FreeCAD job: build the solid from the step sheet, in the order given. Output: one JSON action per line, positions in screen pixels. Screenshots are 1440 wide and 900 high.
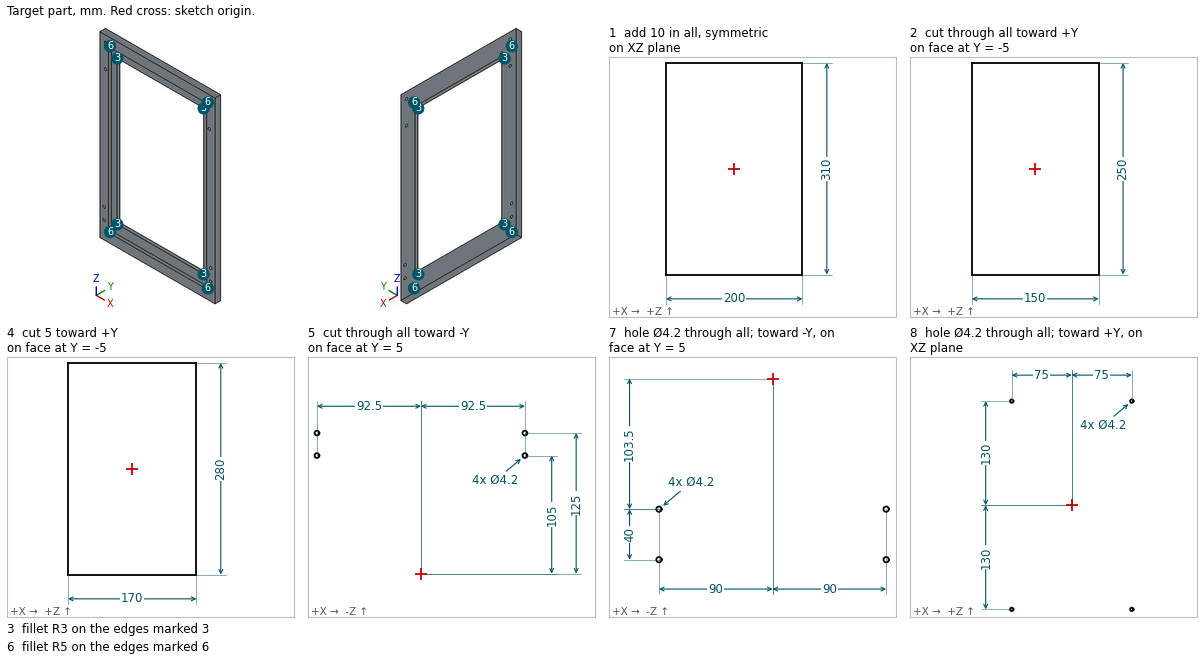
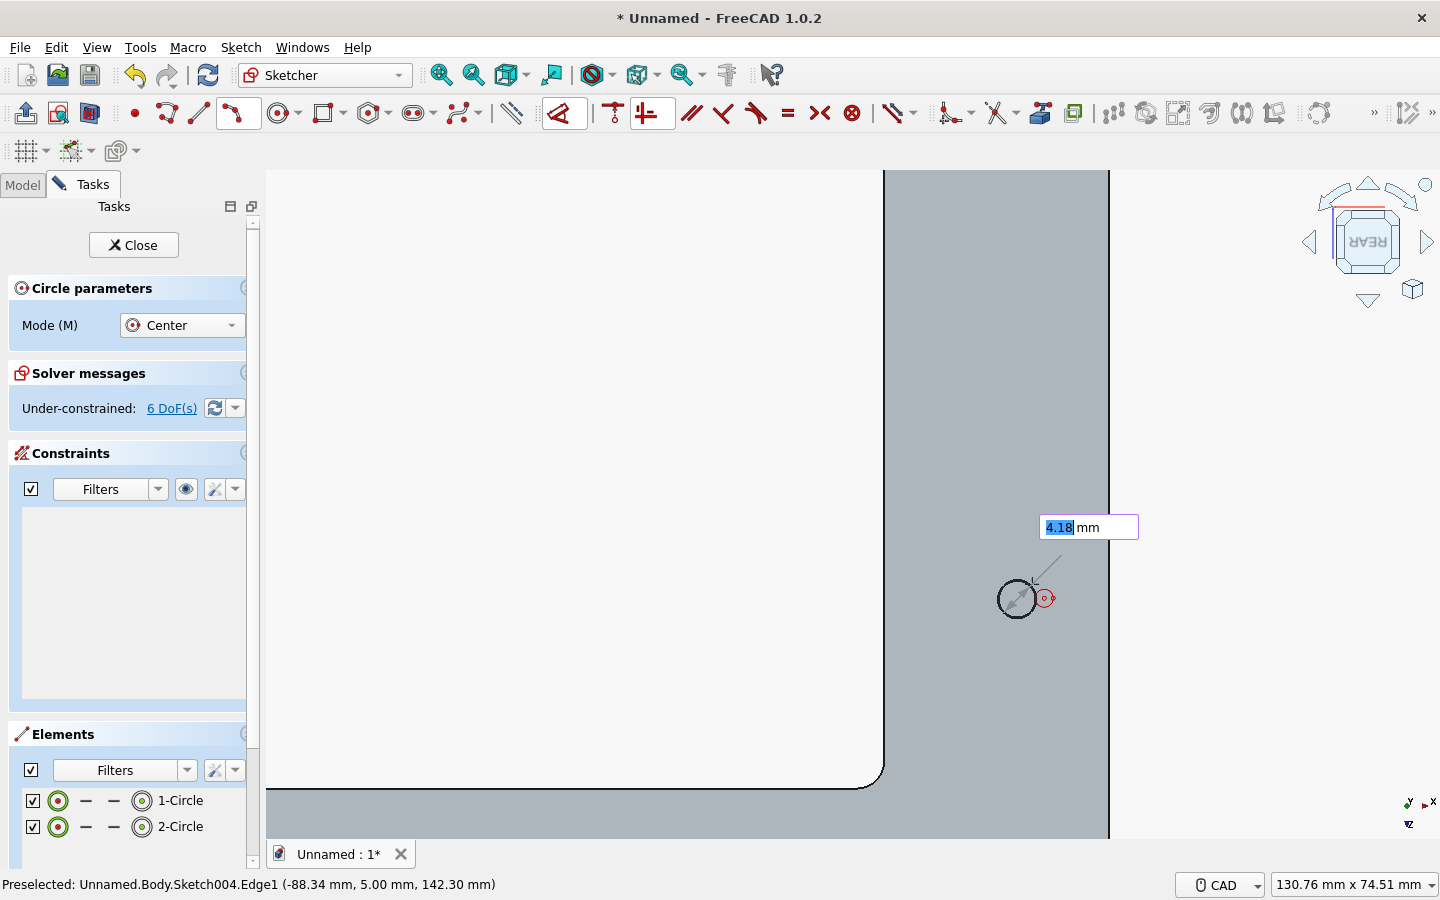
{"action": "left_click", "coordinate": [1032, 582]}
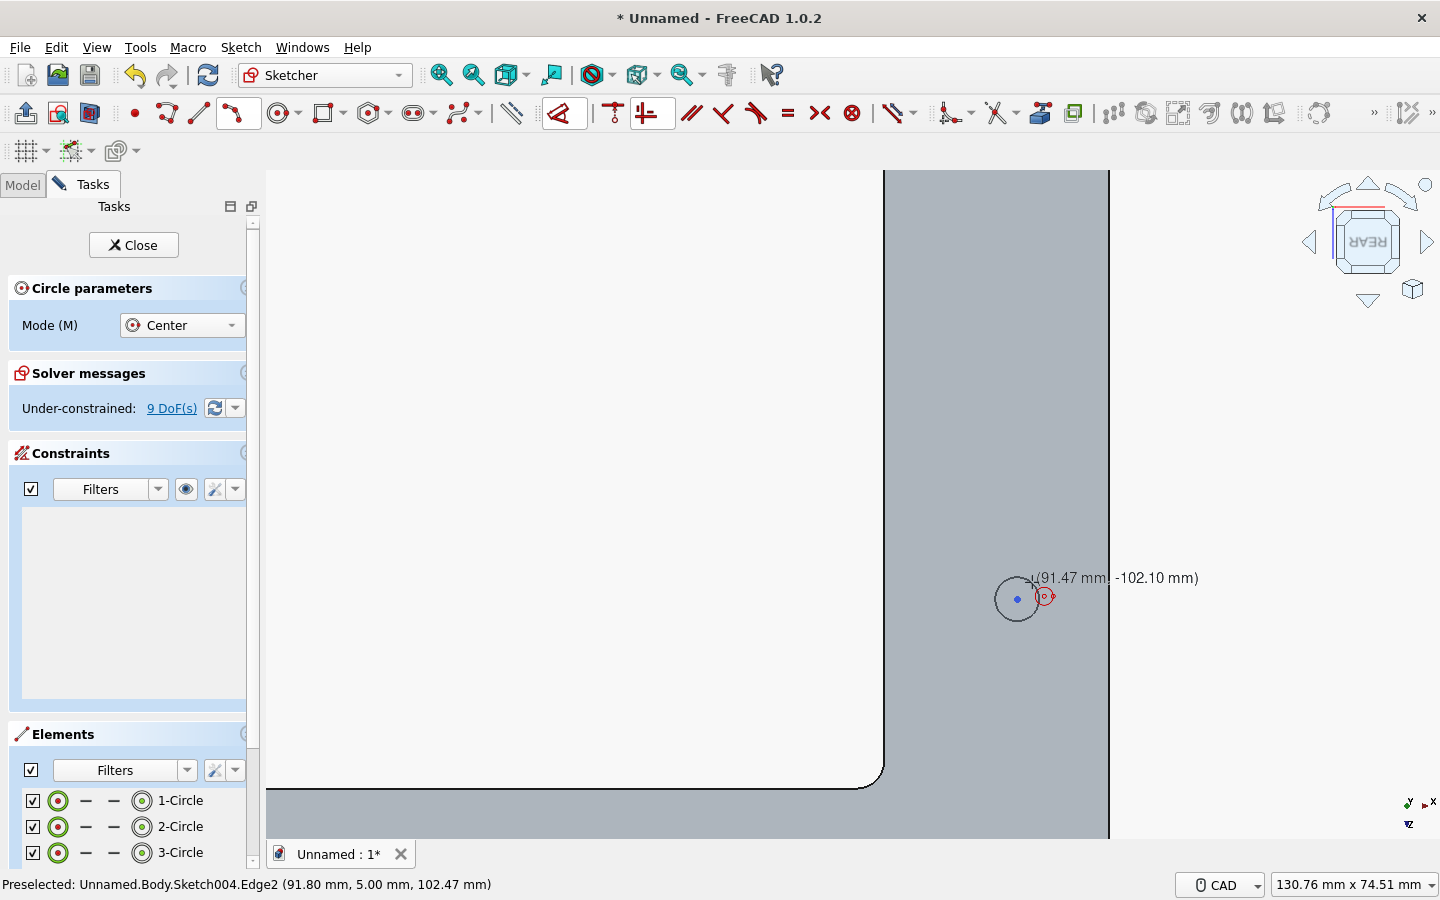
{"action": "scroll", "coordinate": [1032, 584], "scroll_direction": "down", "scroll_amount": 6}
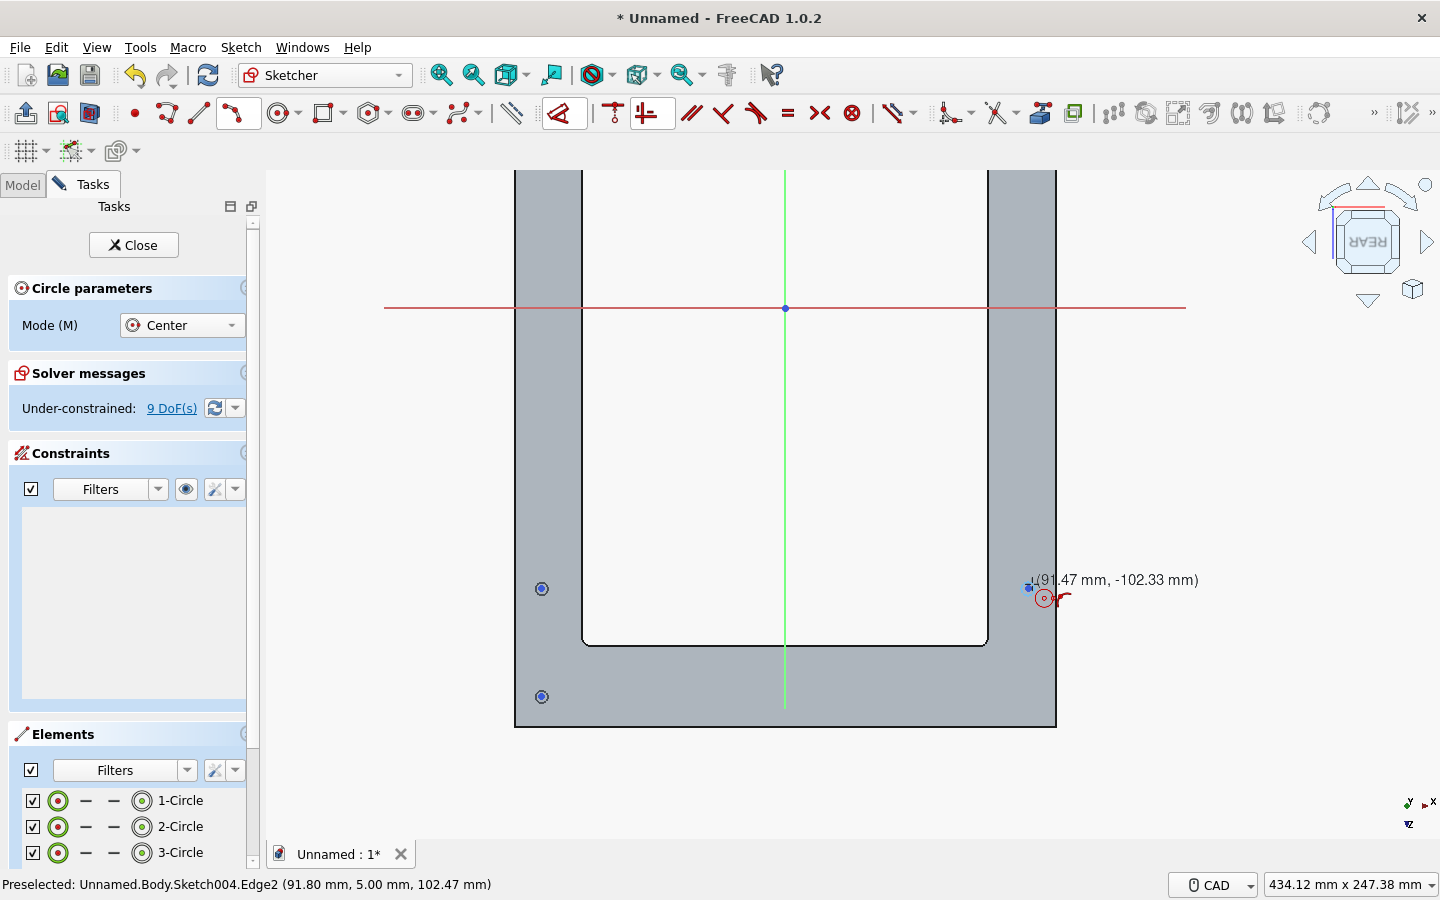
{"action": "scroll", "coordinate": [1028, 696], "scroll_direction": "up", "scroll_amount": 7}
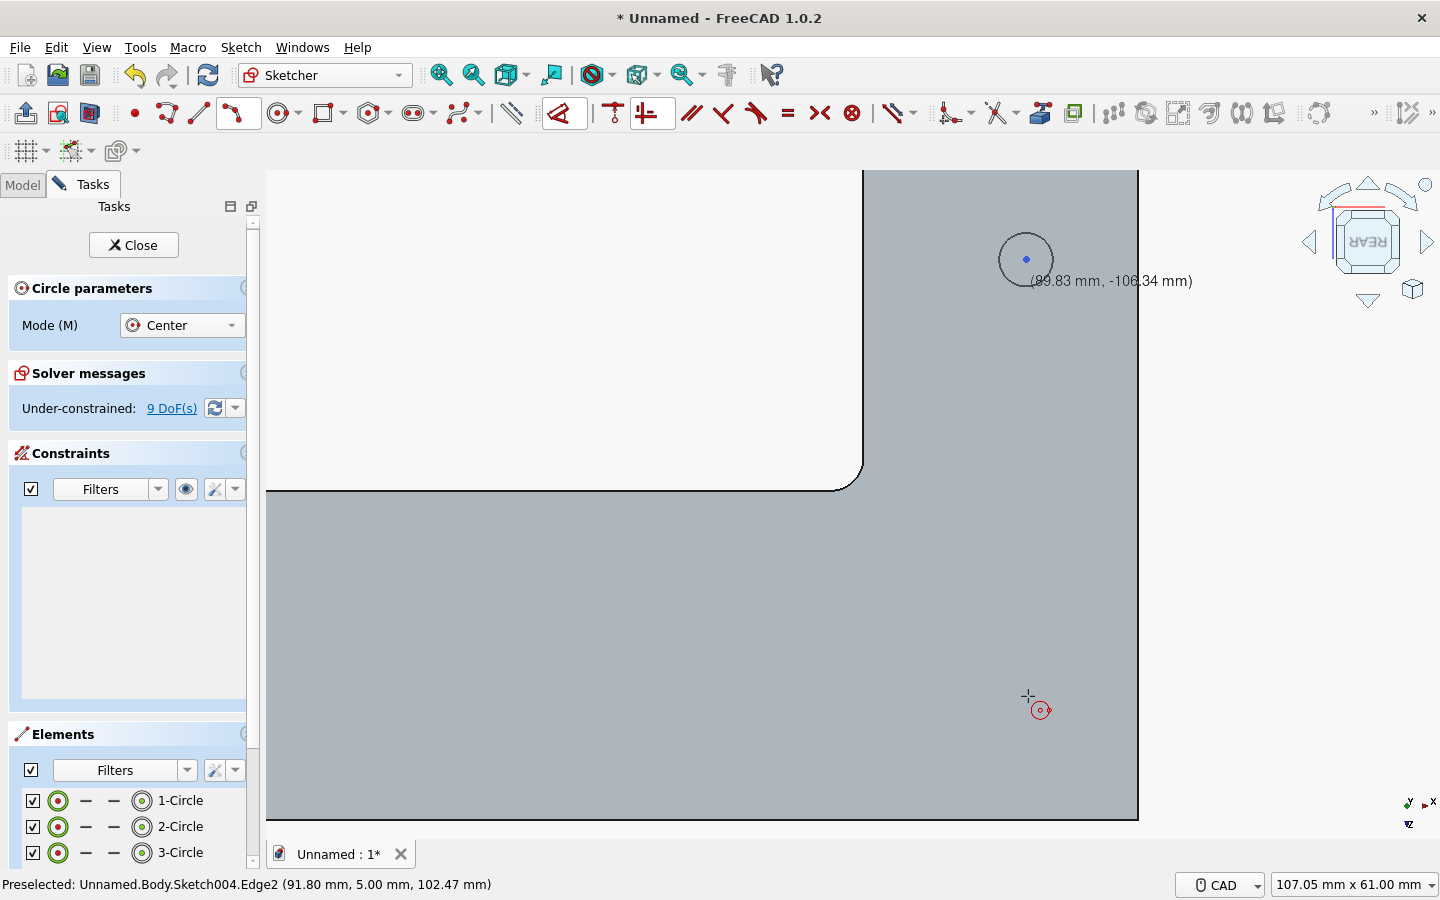
{"action": "scroll", "coordinate": [1028, 696], "scroll_direction": "down", "scroll_amount": 7}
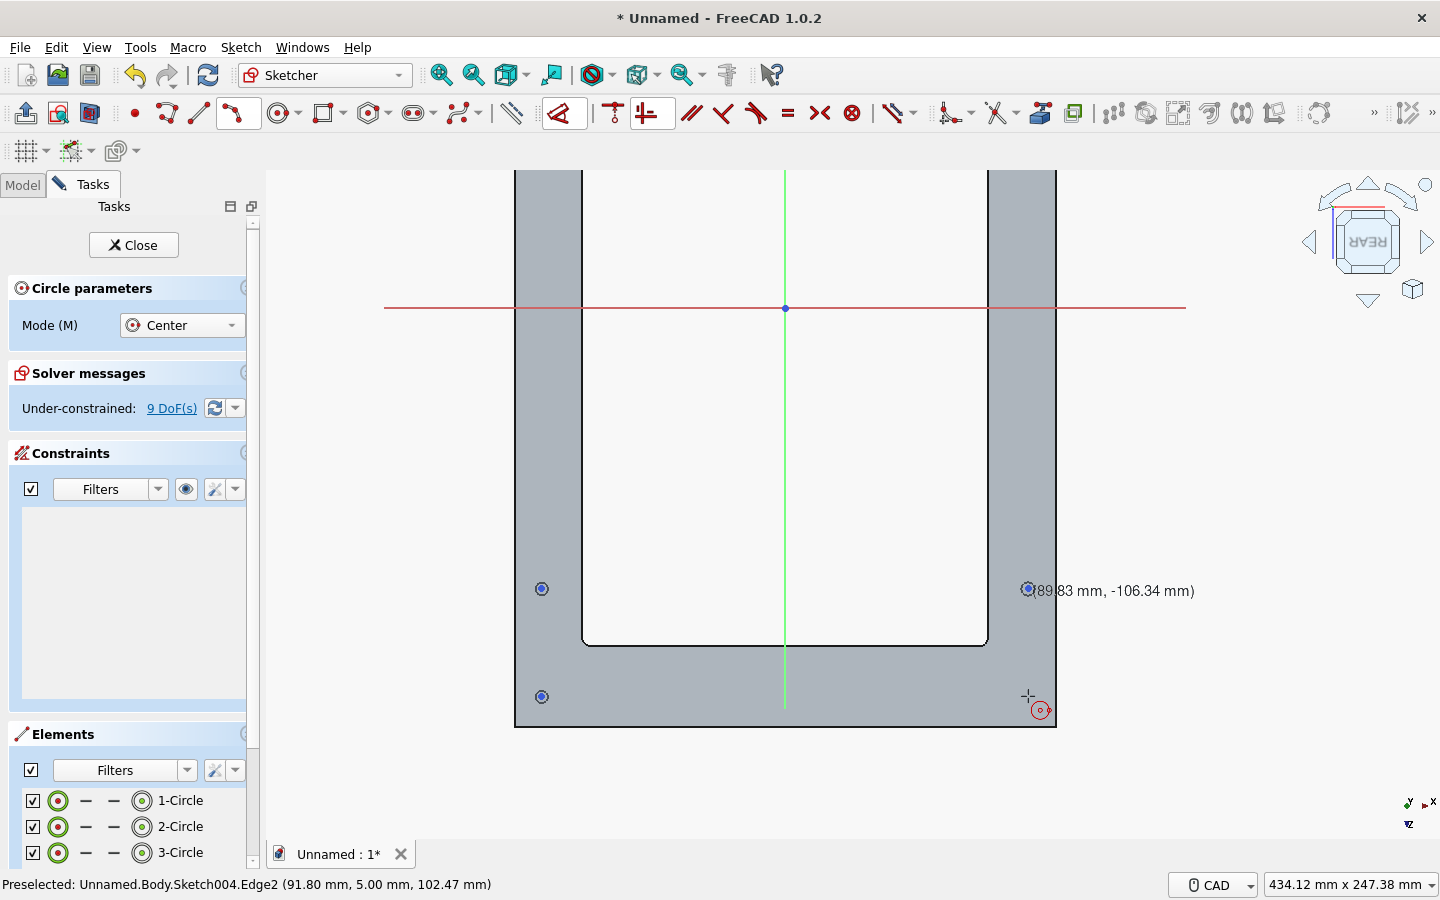
{"action": "left_click", "coordinate": [1028, 696]}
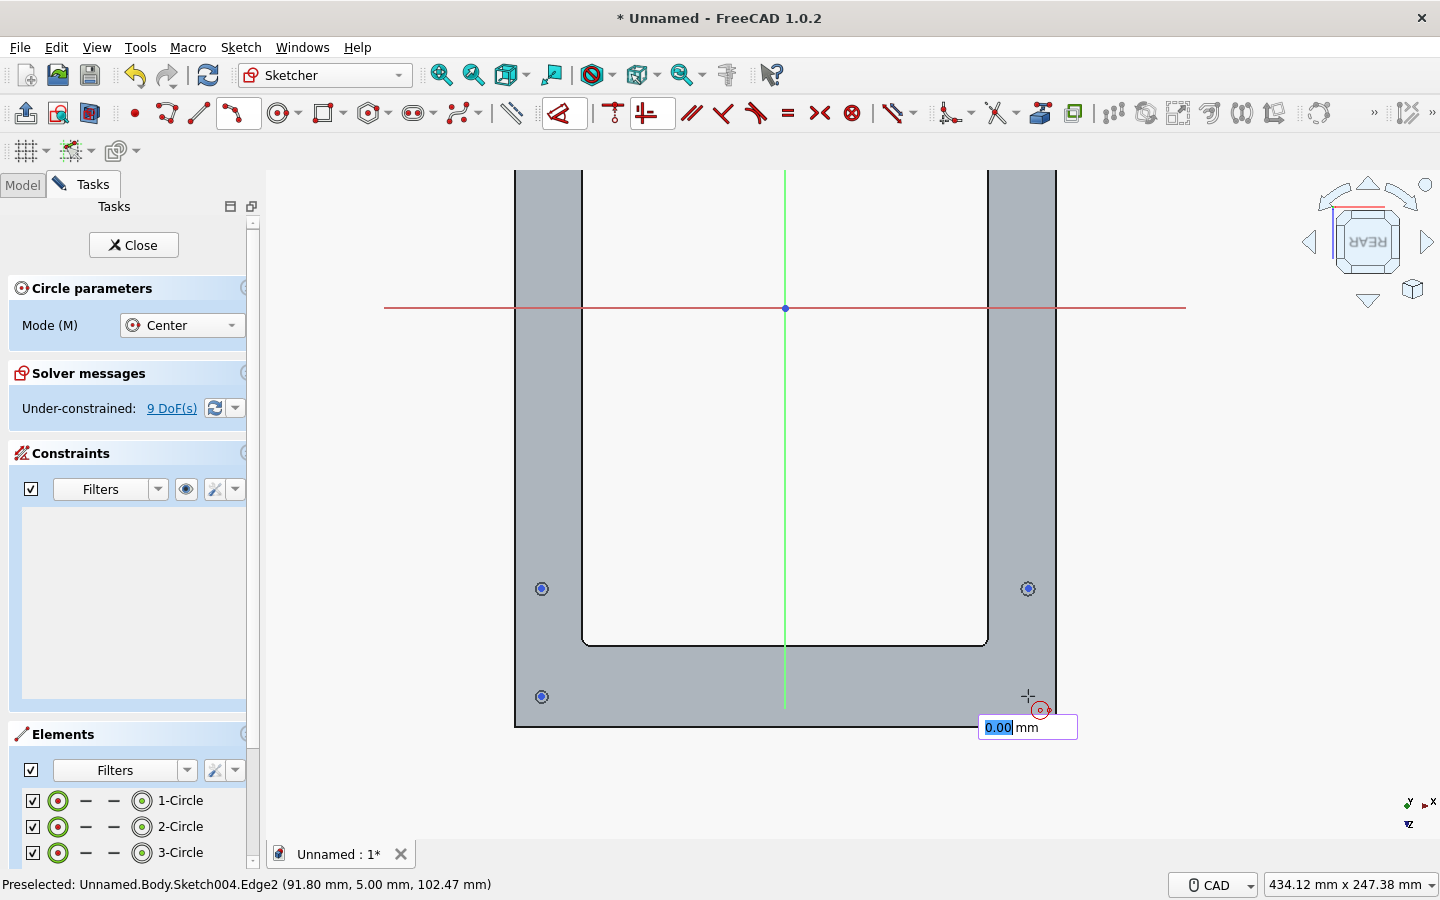
{"action": "scroll", "coordinate": [1032, 692], "scroll_direction": "up", "scroll_amount": 6}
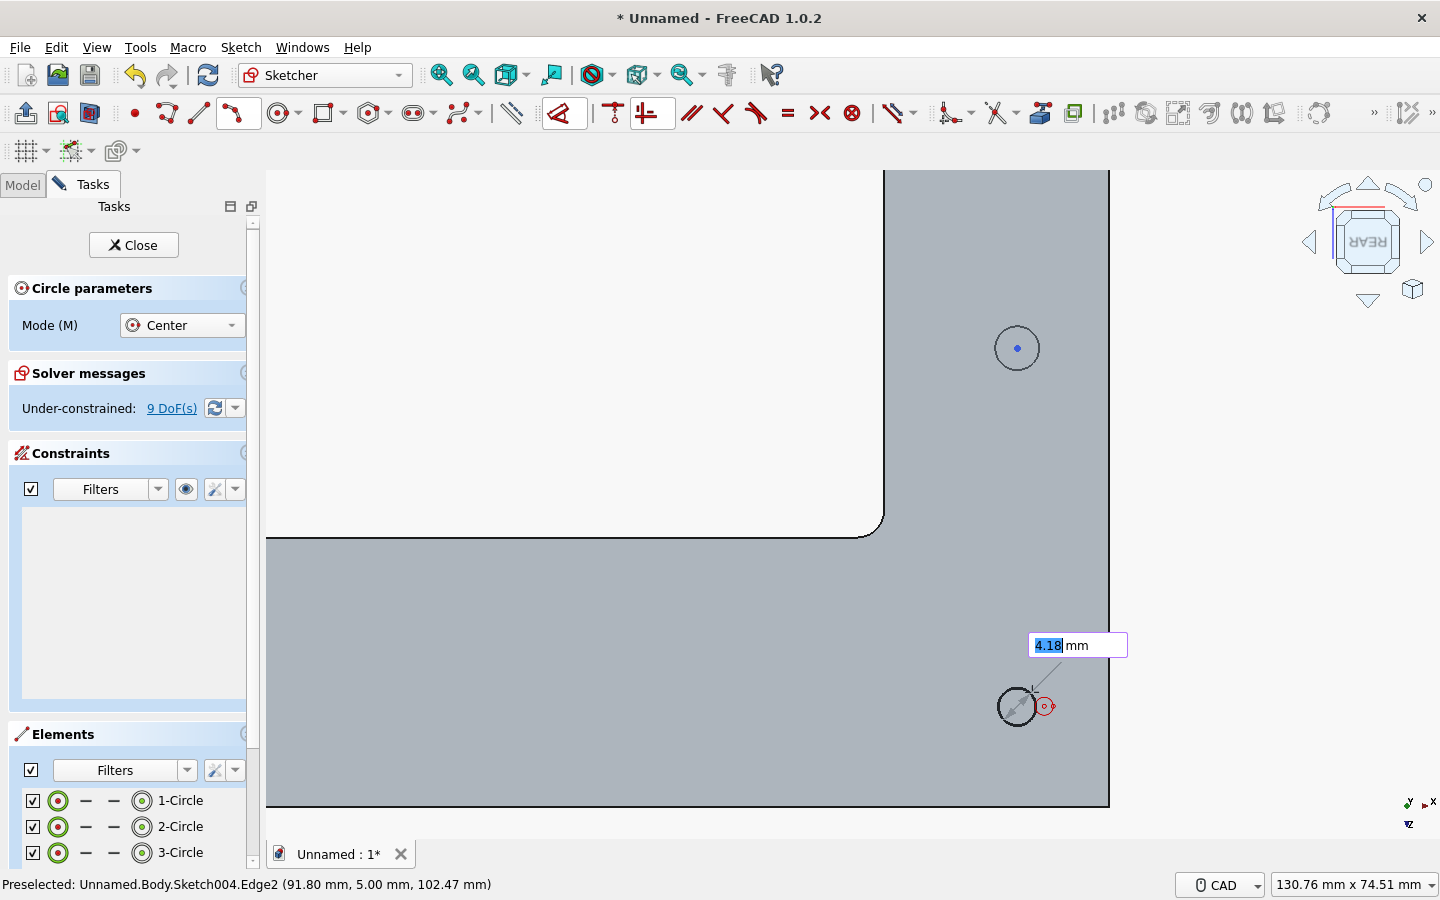
{"action": "left_click", "coordinate": [1032, 690]}
{"action": "key", "text": "Escape"}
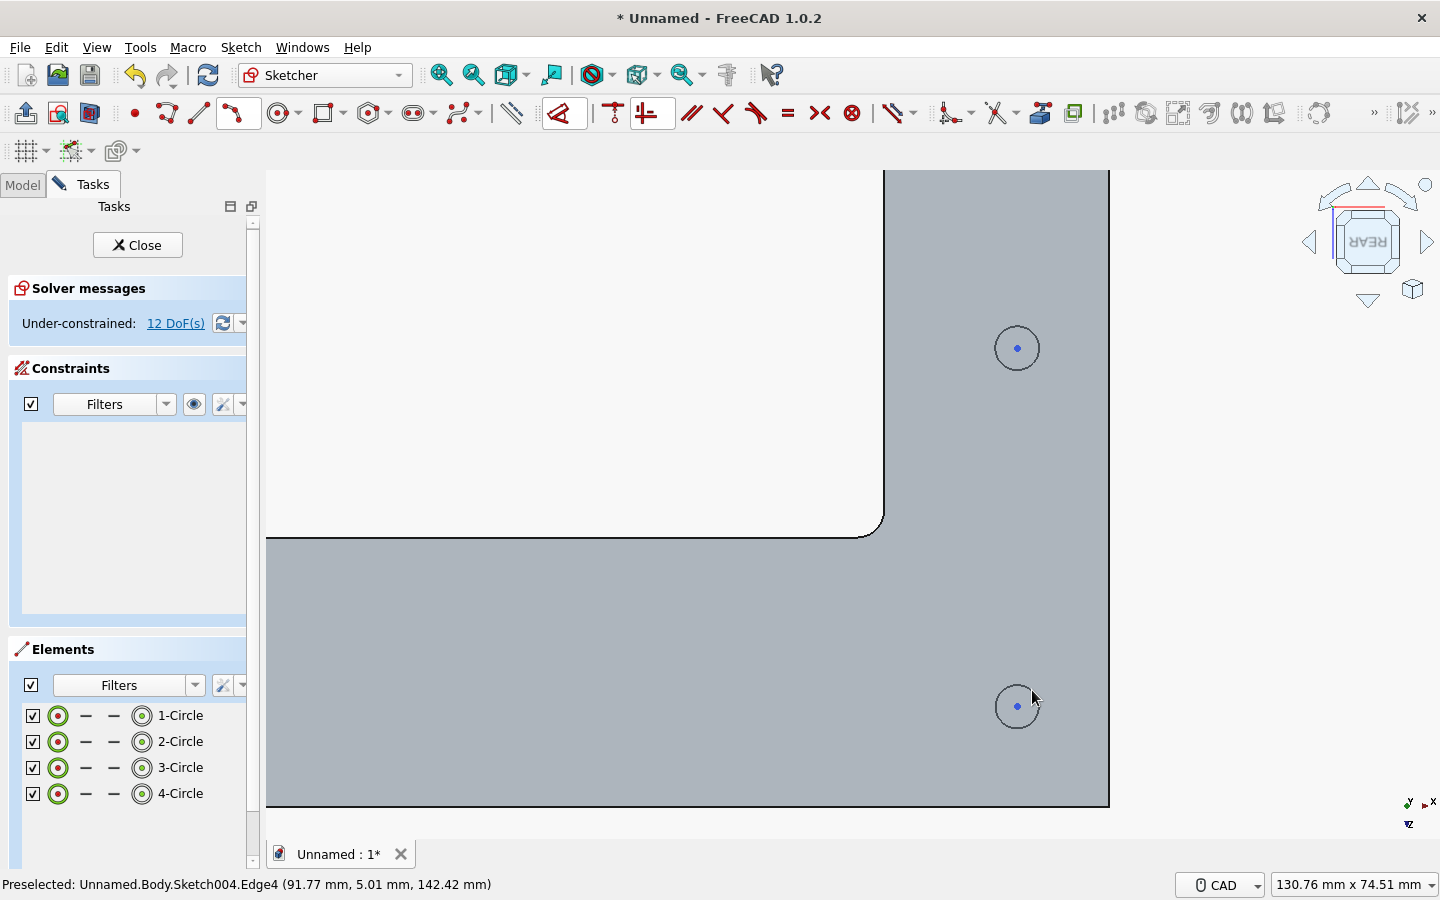
{"action": "scroll", "coordinate": [1032, 692], "scroll_direction": "down", "scroll_amount": 6}